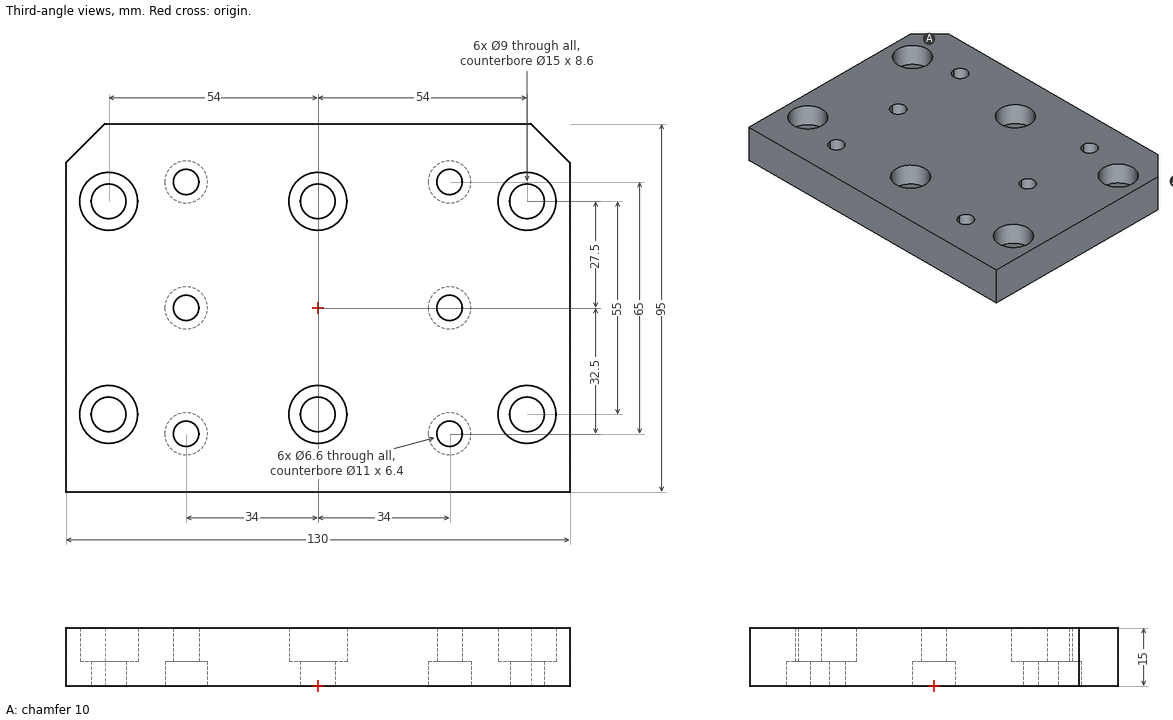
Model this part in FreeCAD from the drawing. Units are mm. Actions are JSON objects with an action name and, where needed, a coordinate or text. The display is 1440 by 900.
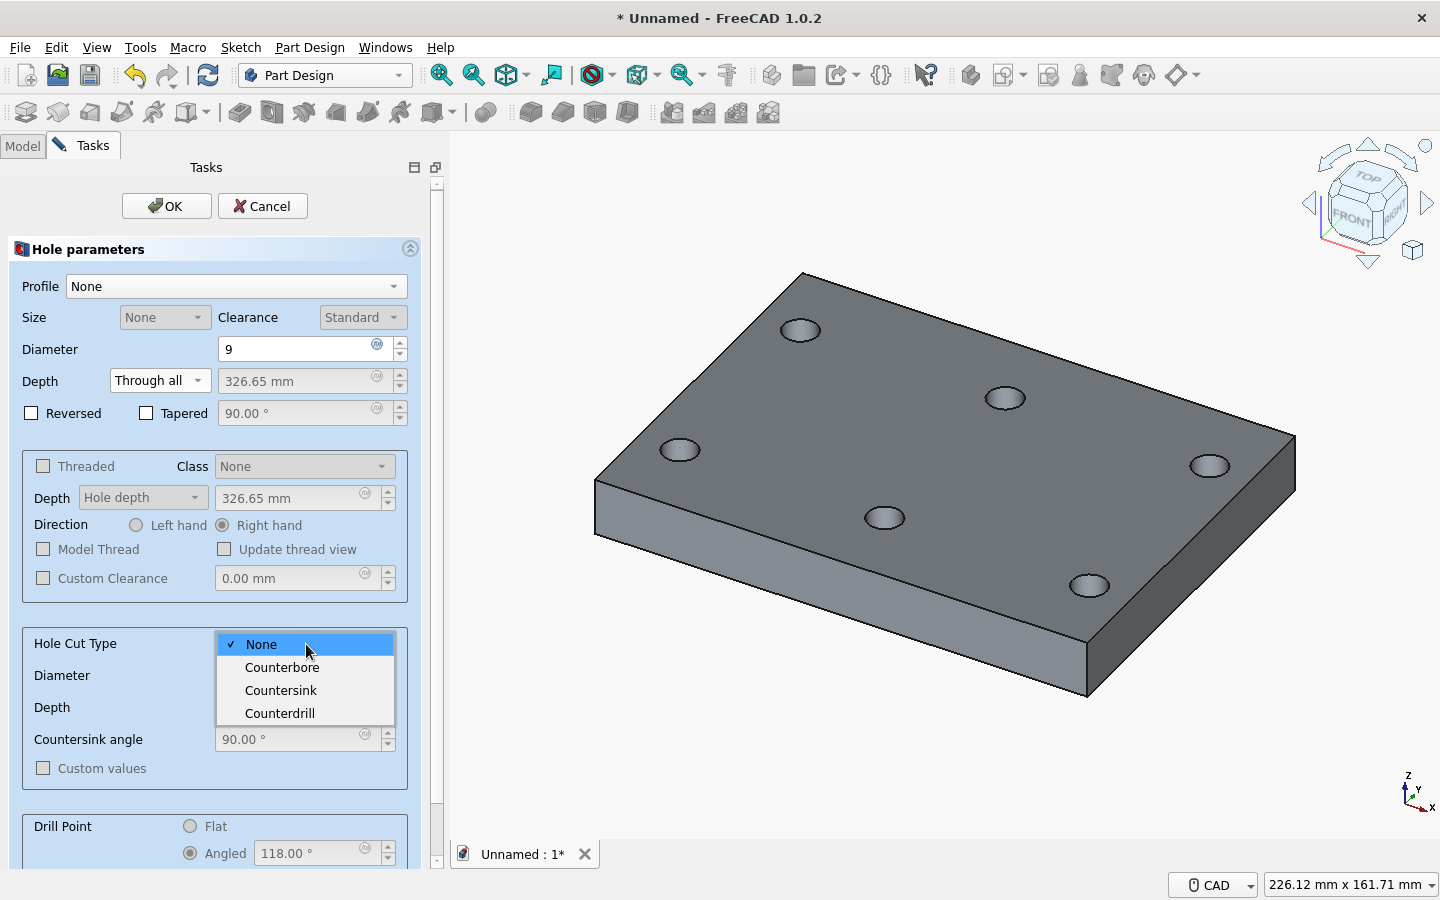
{"action": "left_click", "coordinate": [304, 668]}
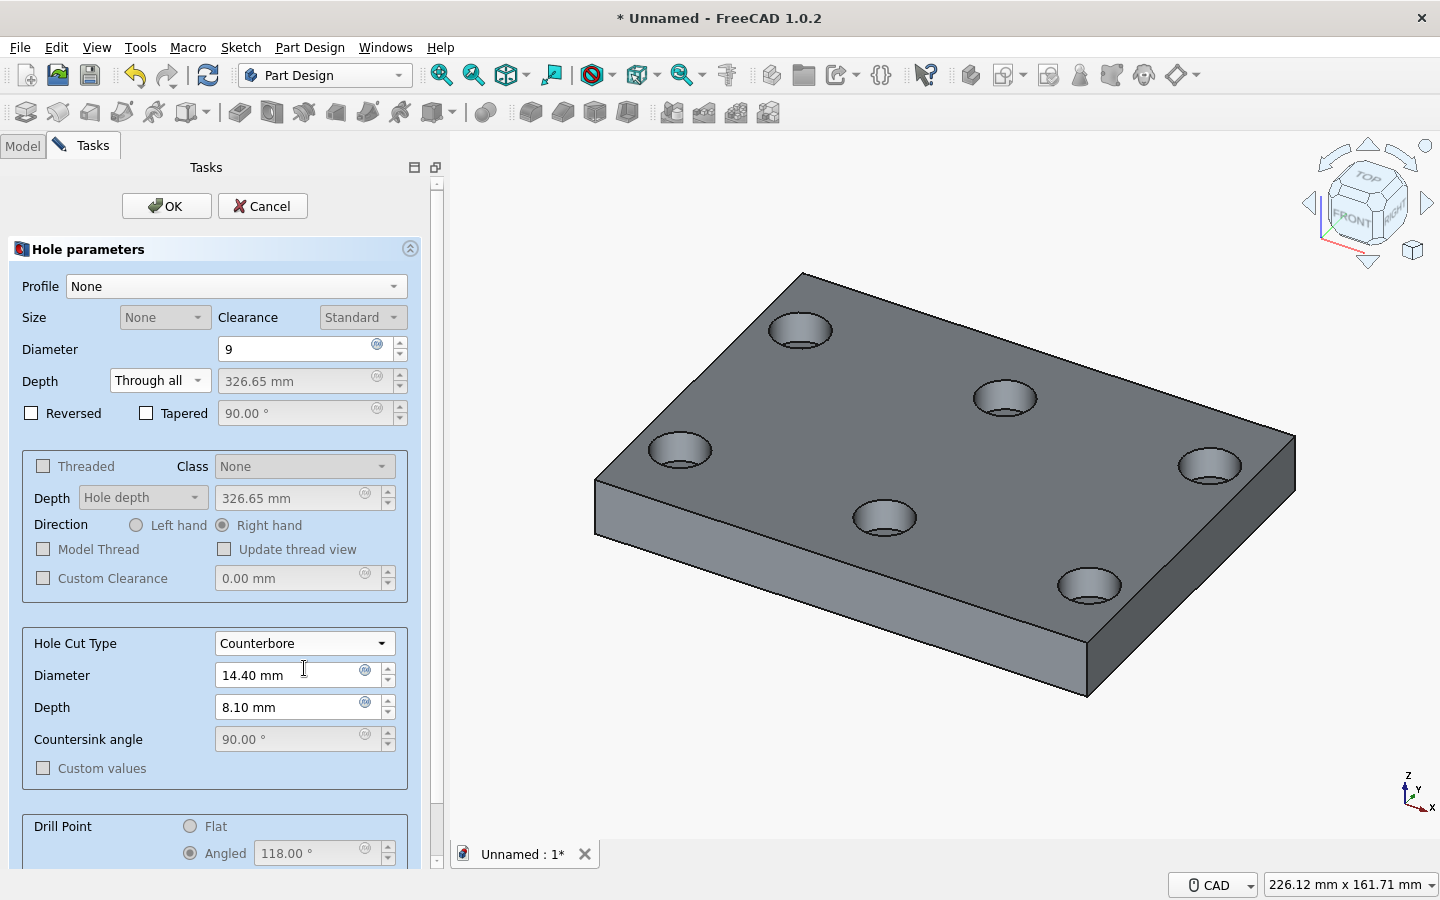
{"action": "triple_click", "coordinate": [298, 675]}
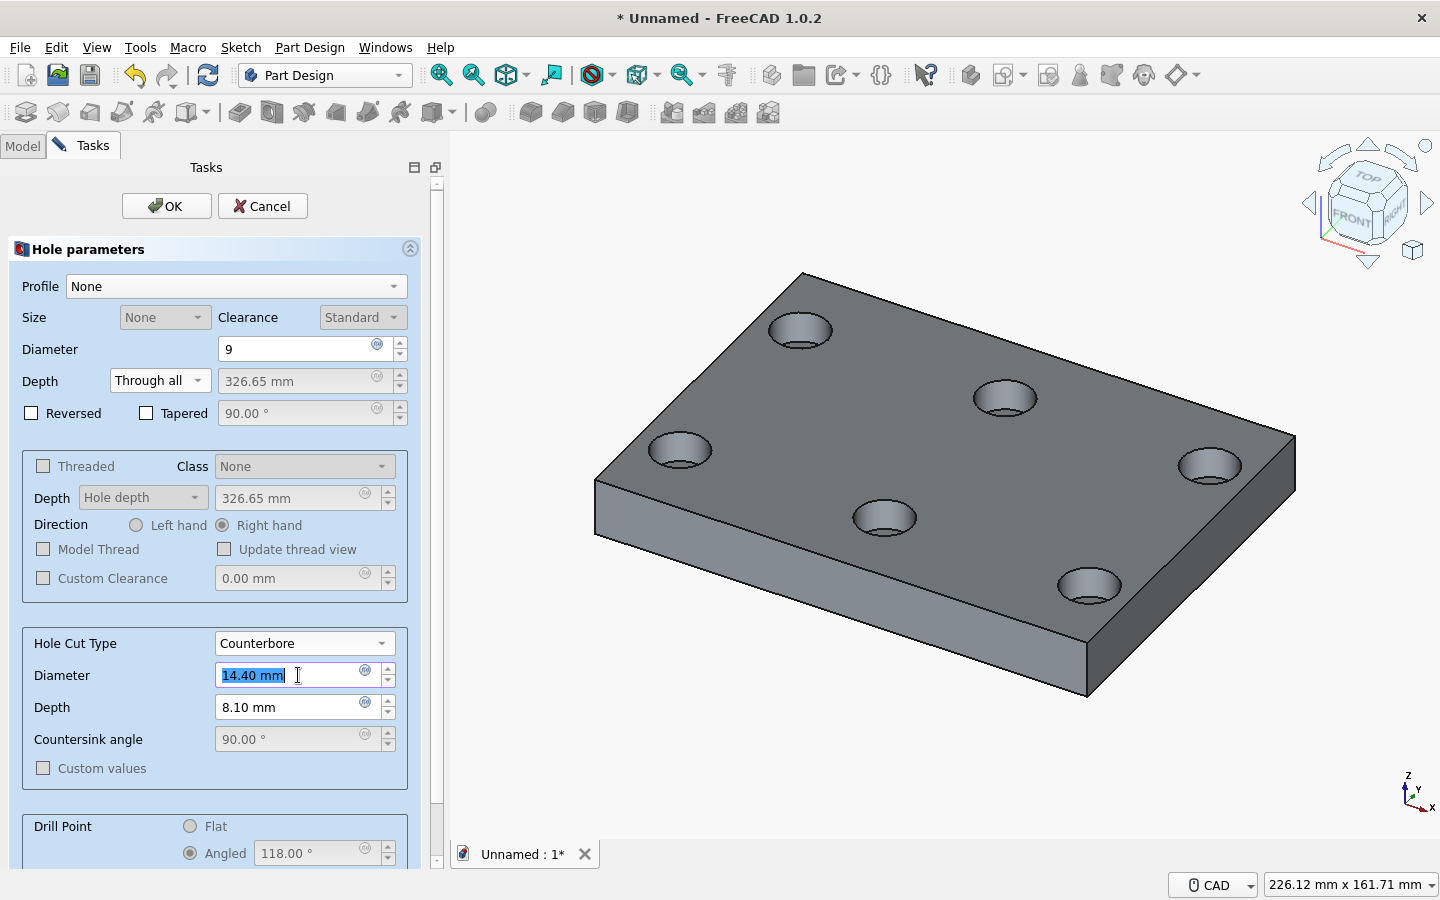
{"action": "type", "text": "15"}
{"action": "key", "text": "Tab"}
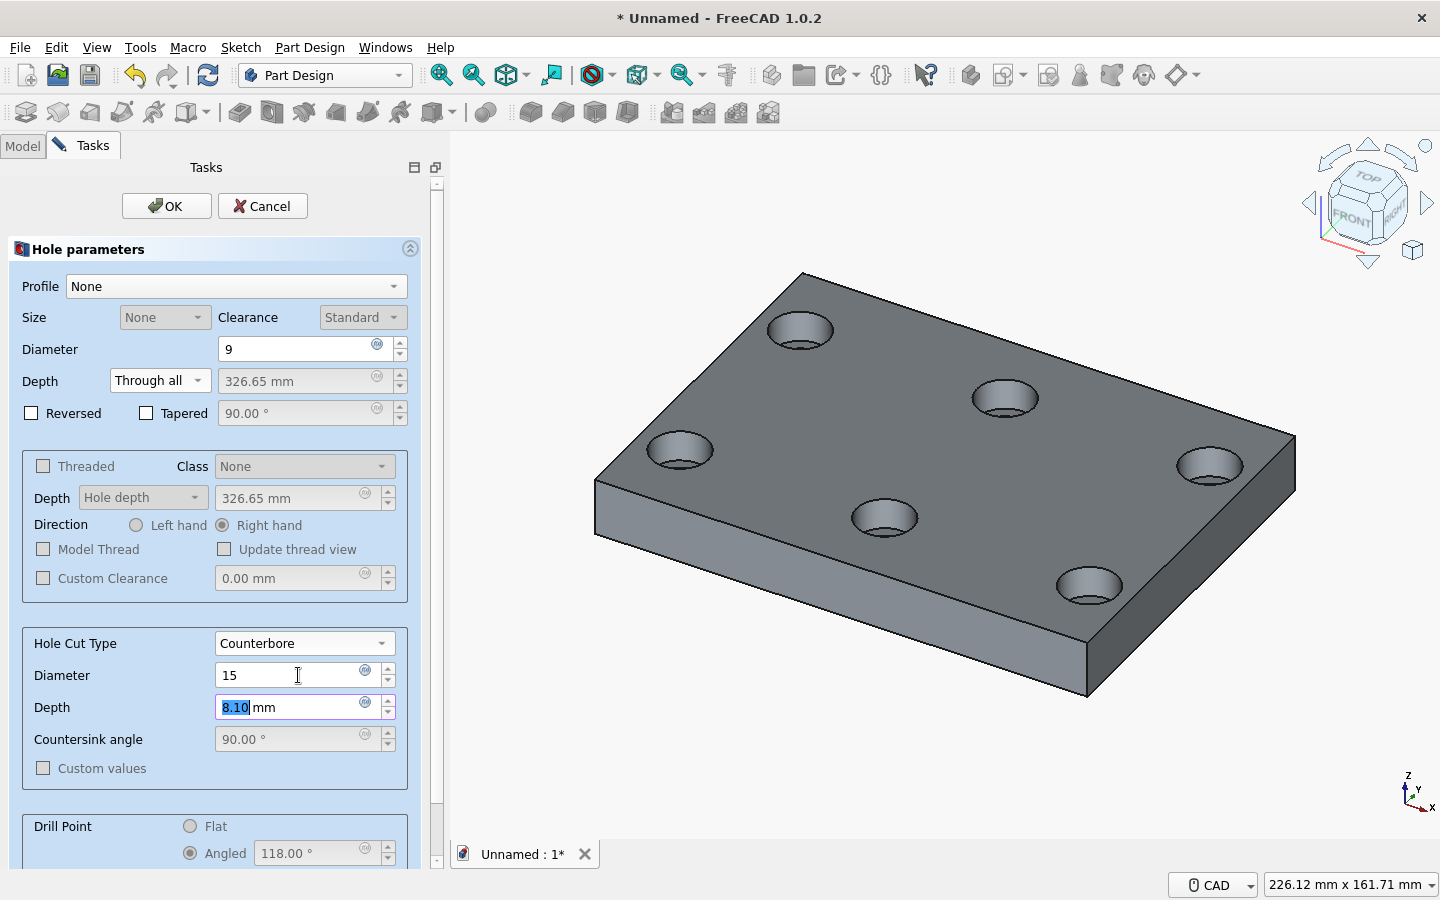
{"action": "type", "text": "8.6"}
{"action": "key", "text": "Tab"}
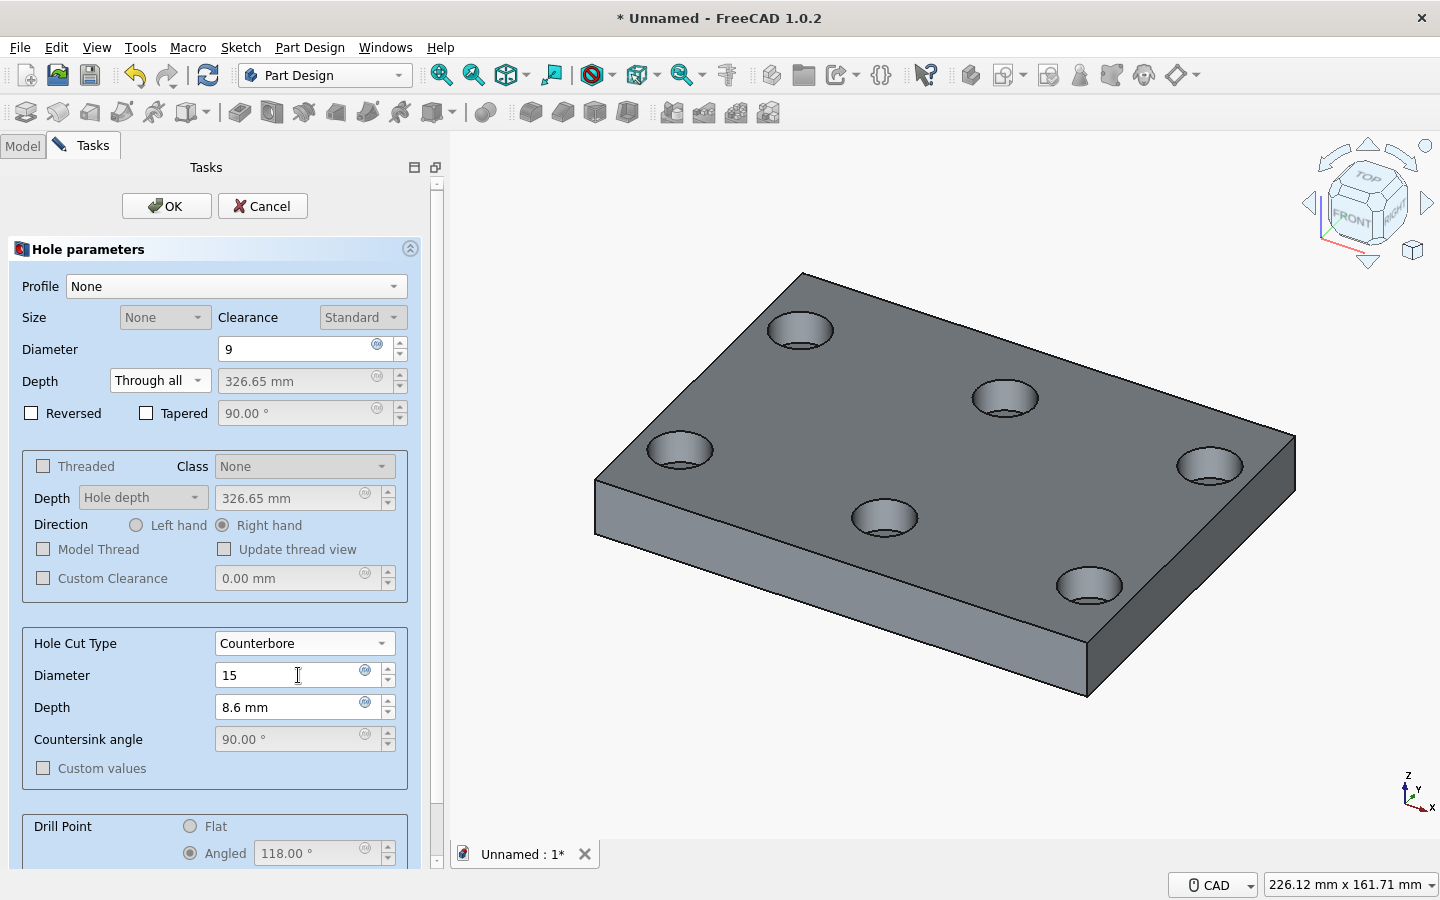
{"action": "left_click", "coordinate": [167, 206]}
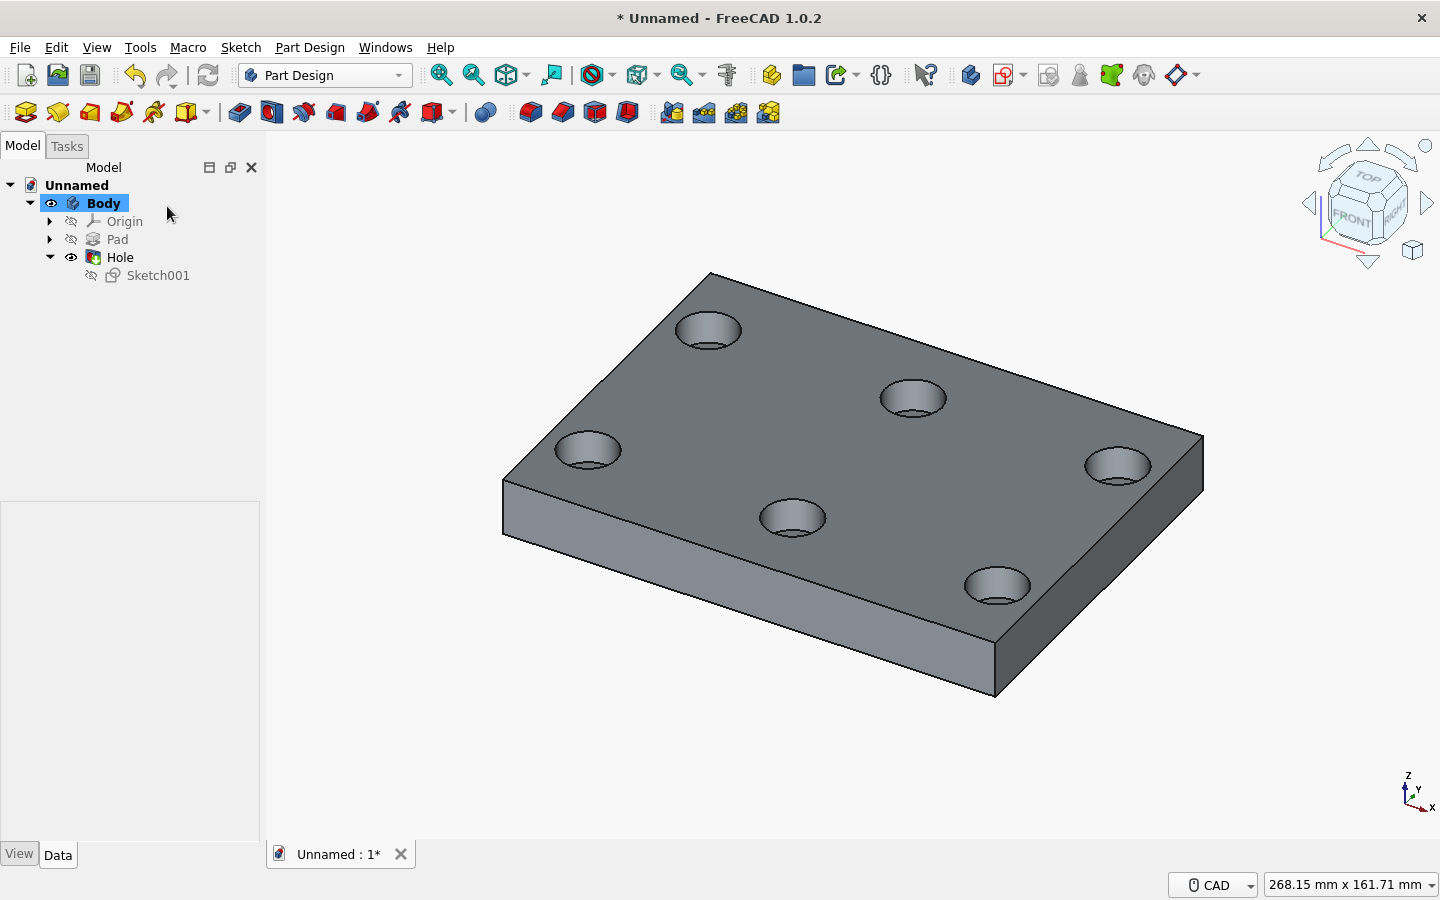
{"action": "key", "text": "0"}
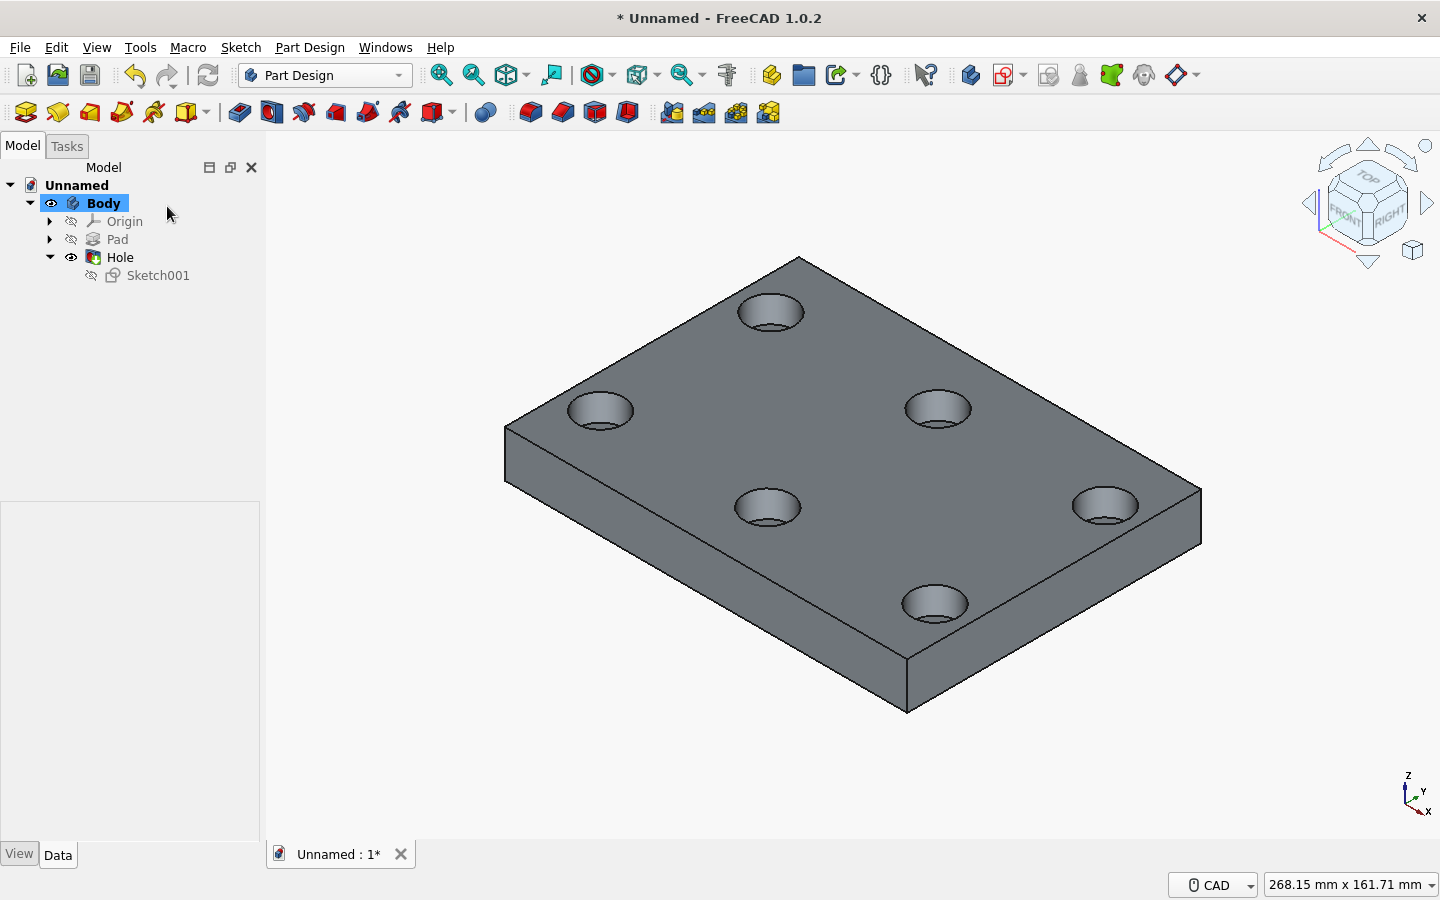
{"action": "key", "text": "2"}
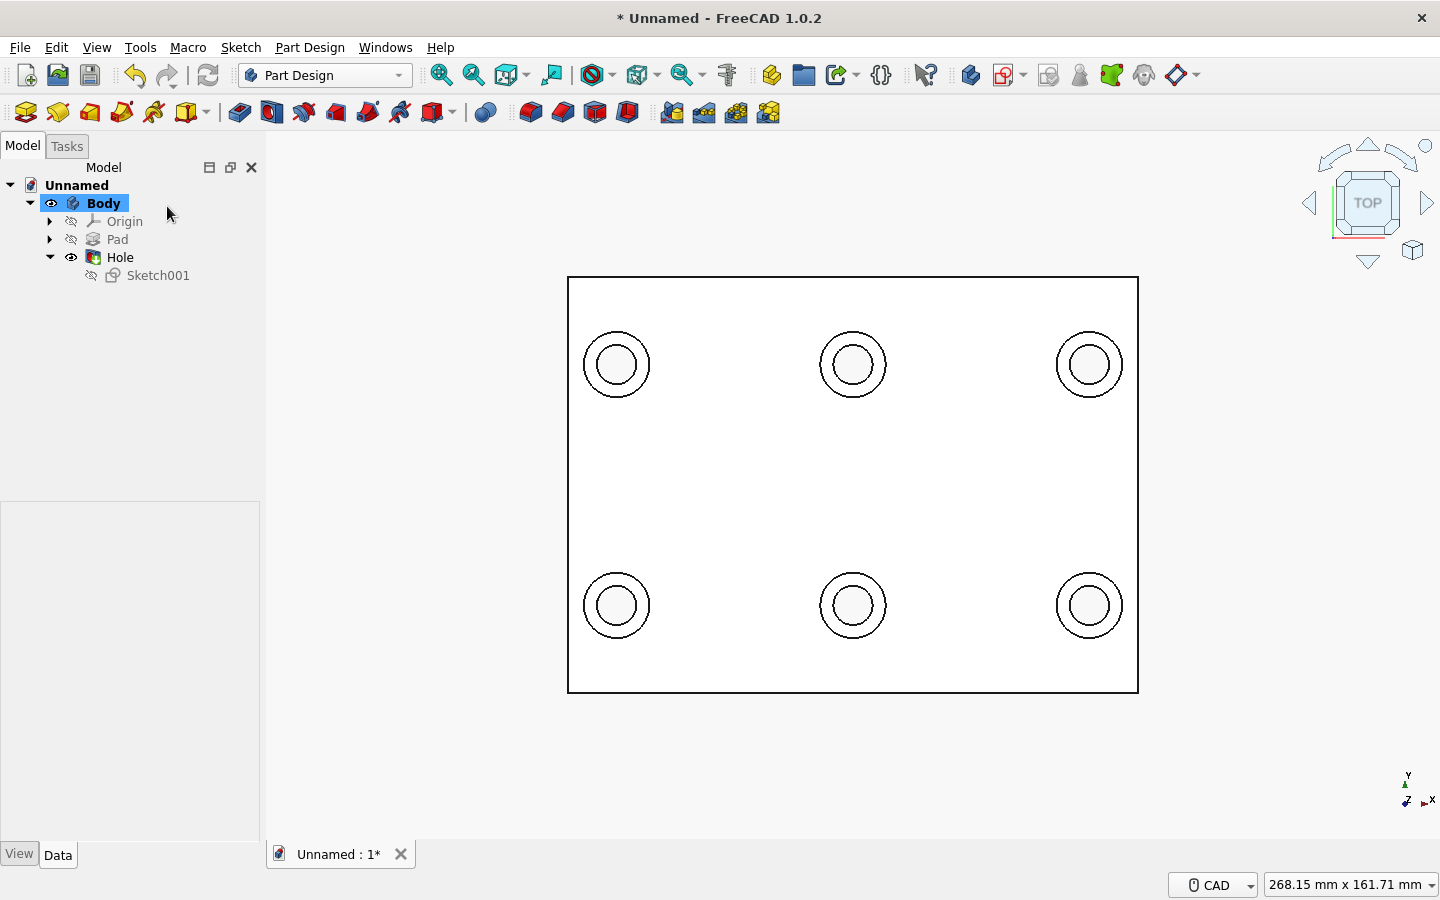
{"action": "key", "text": "1"}